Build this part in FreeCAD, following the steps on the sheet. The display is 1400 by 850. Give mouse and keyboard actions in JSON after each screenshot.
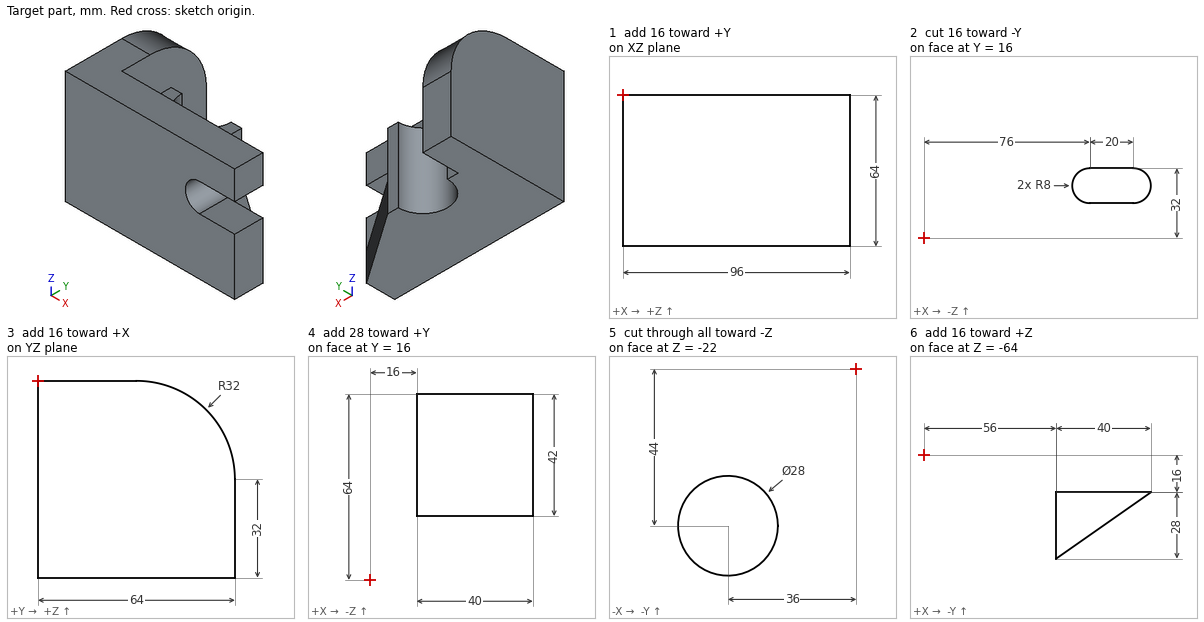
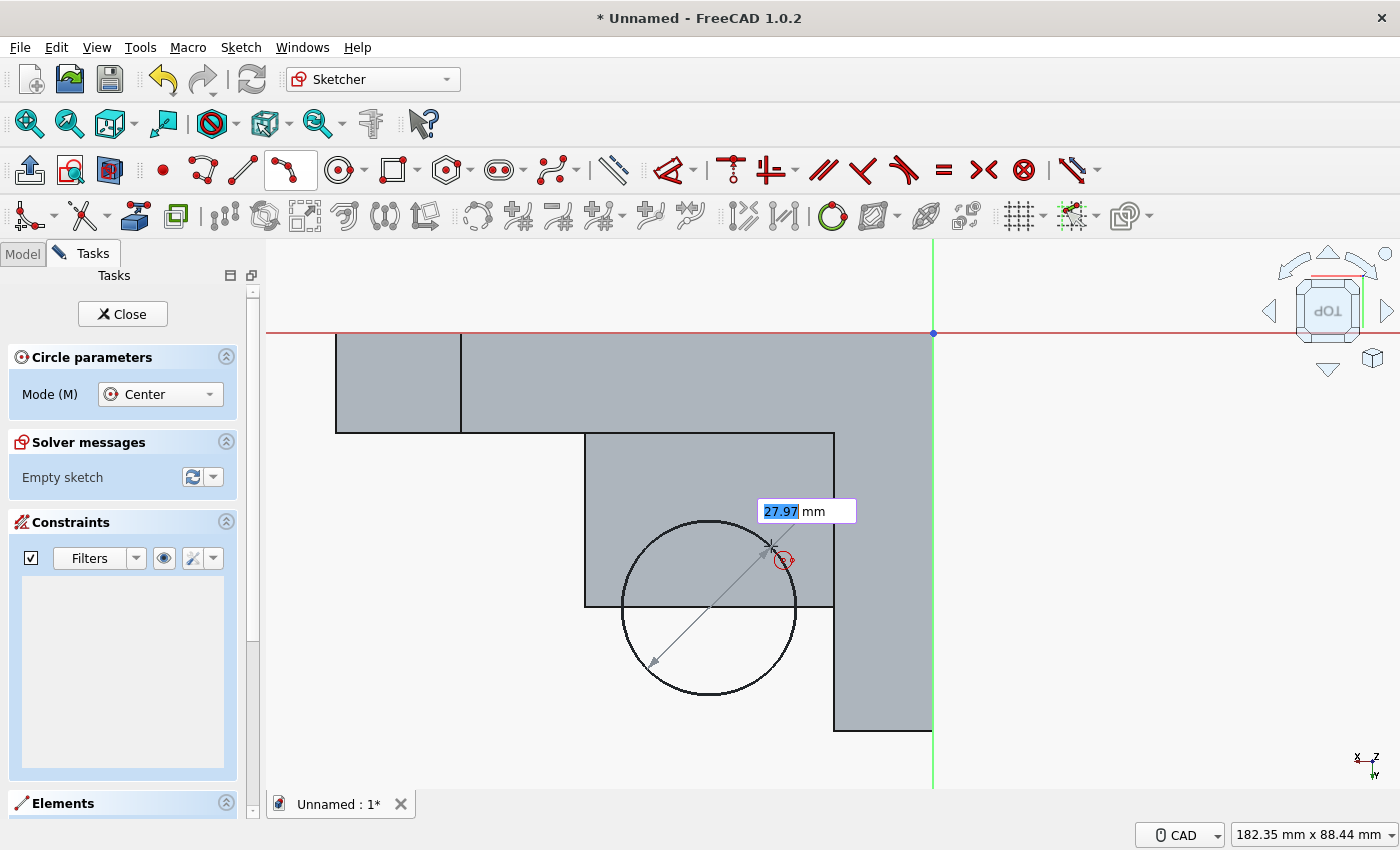
{"action": "type", "text": "28"}
{"action": "key", "text": "Return"}
{"action": "key", "text": "Escape"}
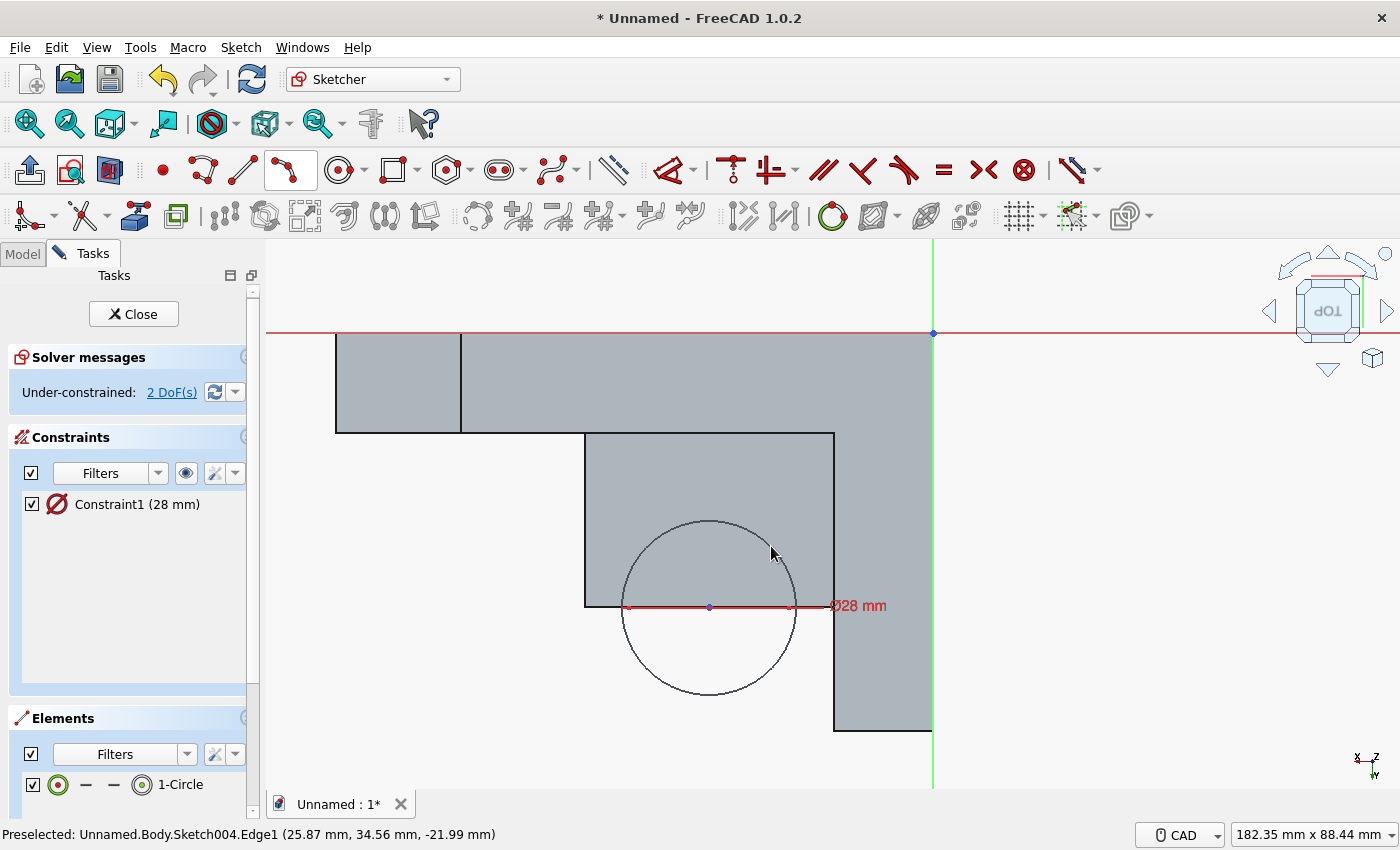
{"action": "key", "text": "d"}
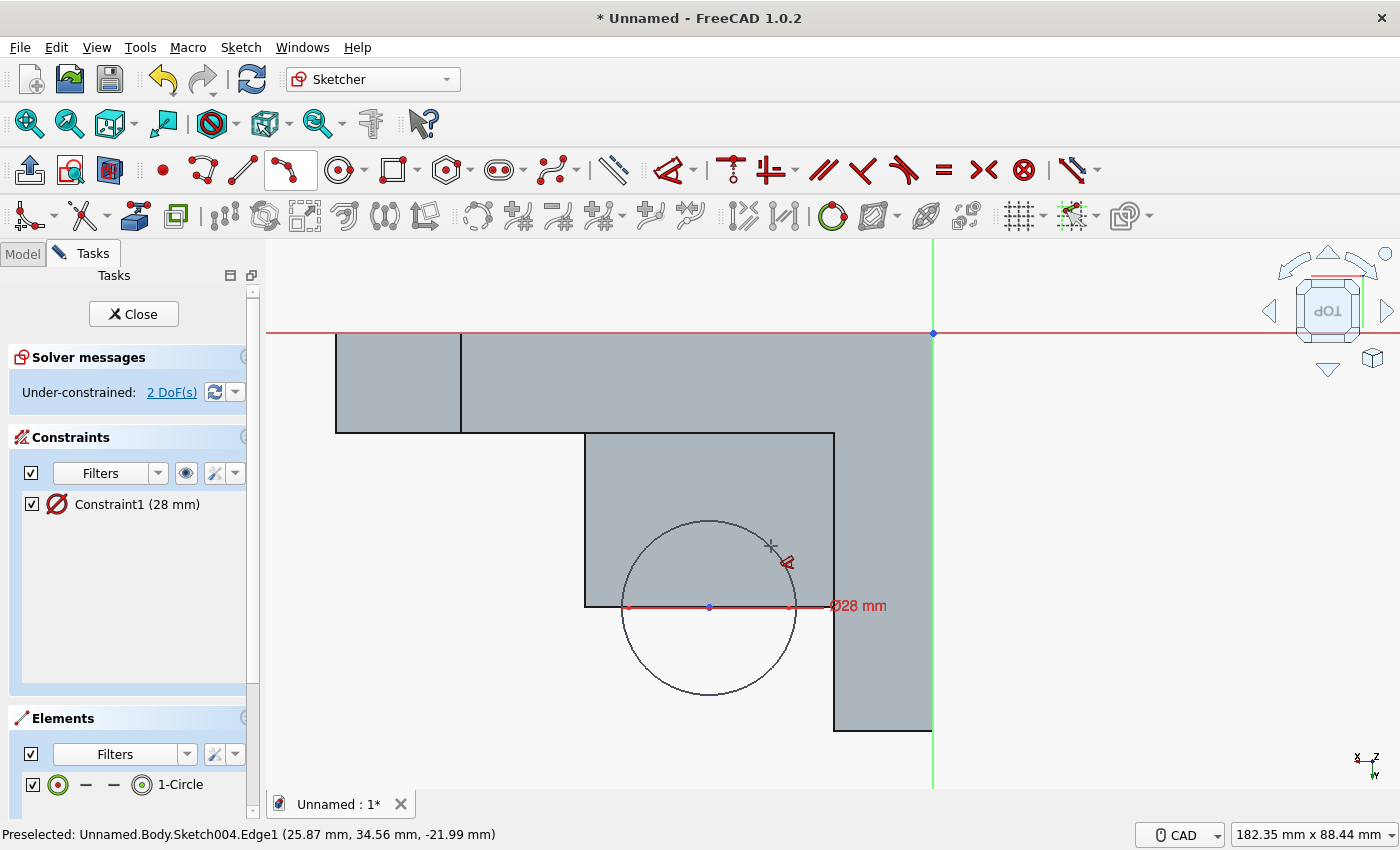
{"action": "left_click", "coordinate": [709, 608]}
{"action": "left_click", "coordinate": [821, 299]}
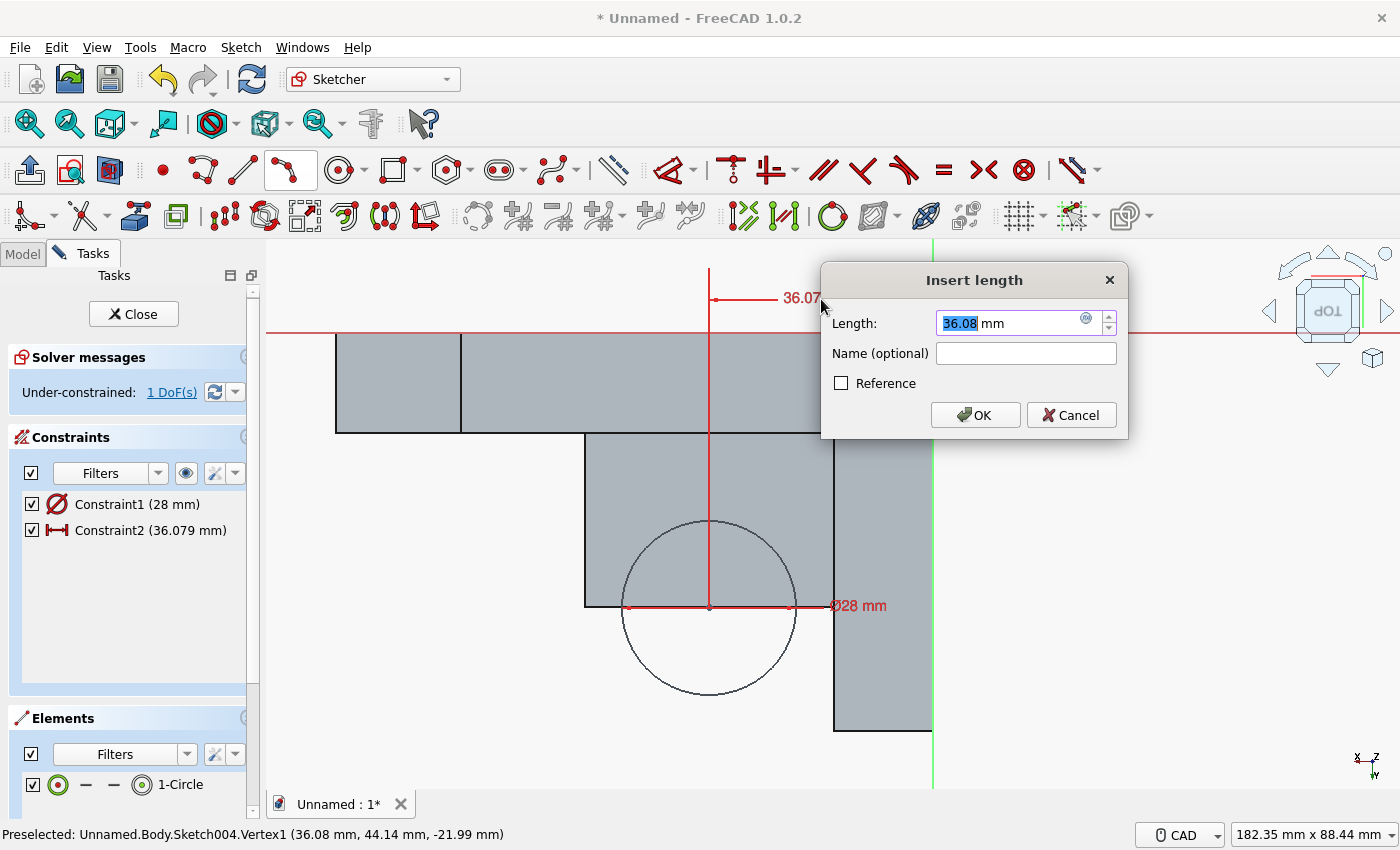
{"action": "type", "text": "36"}
{"action": "key", "text": "Return"}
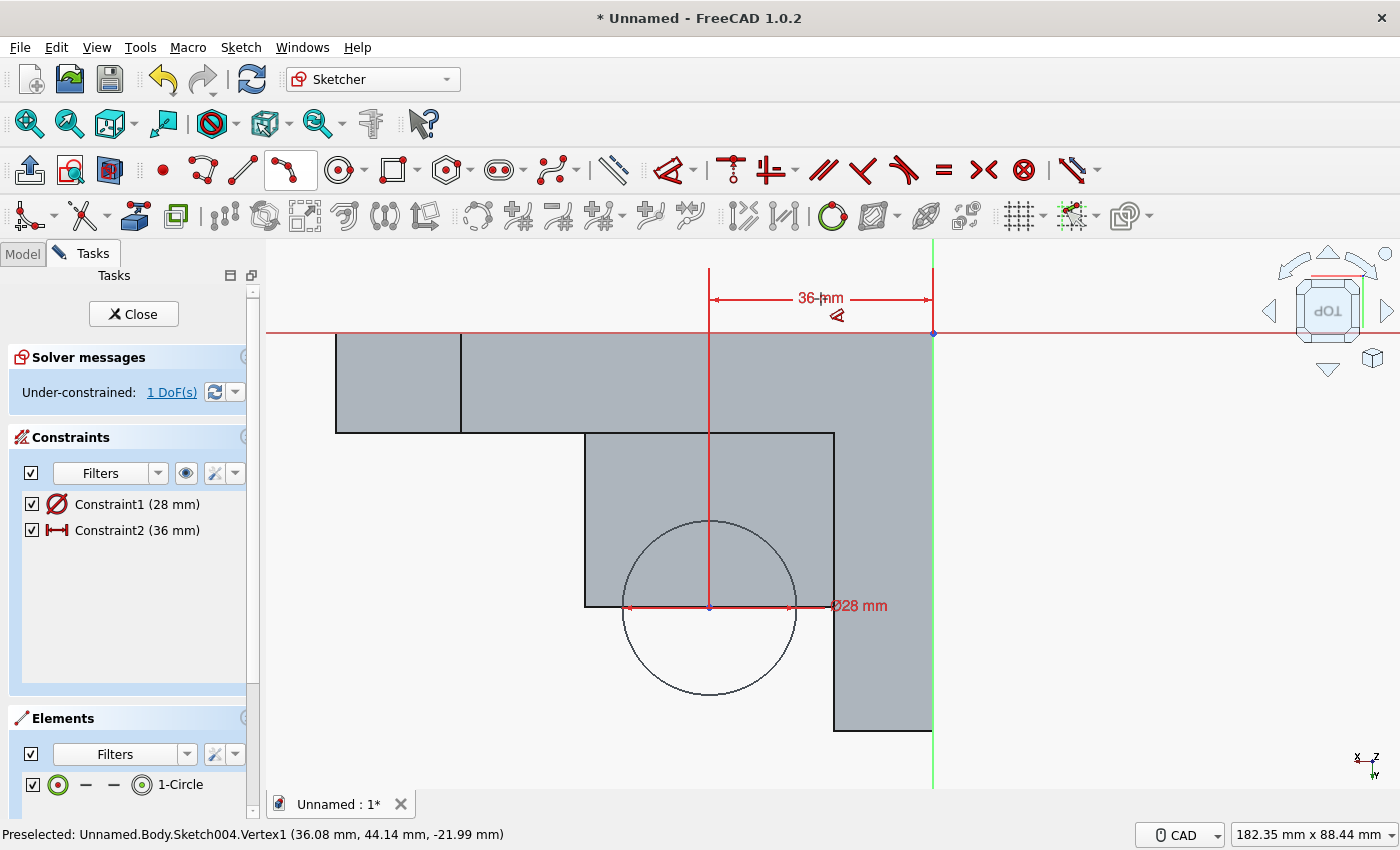
{"action": "left_click", "coordinate": [709, 608]}
{"action": "left_click", "coordinate": [967, 471]}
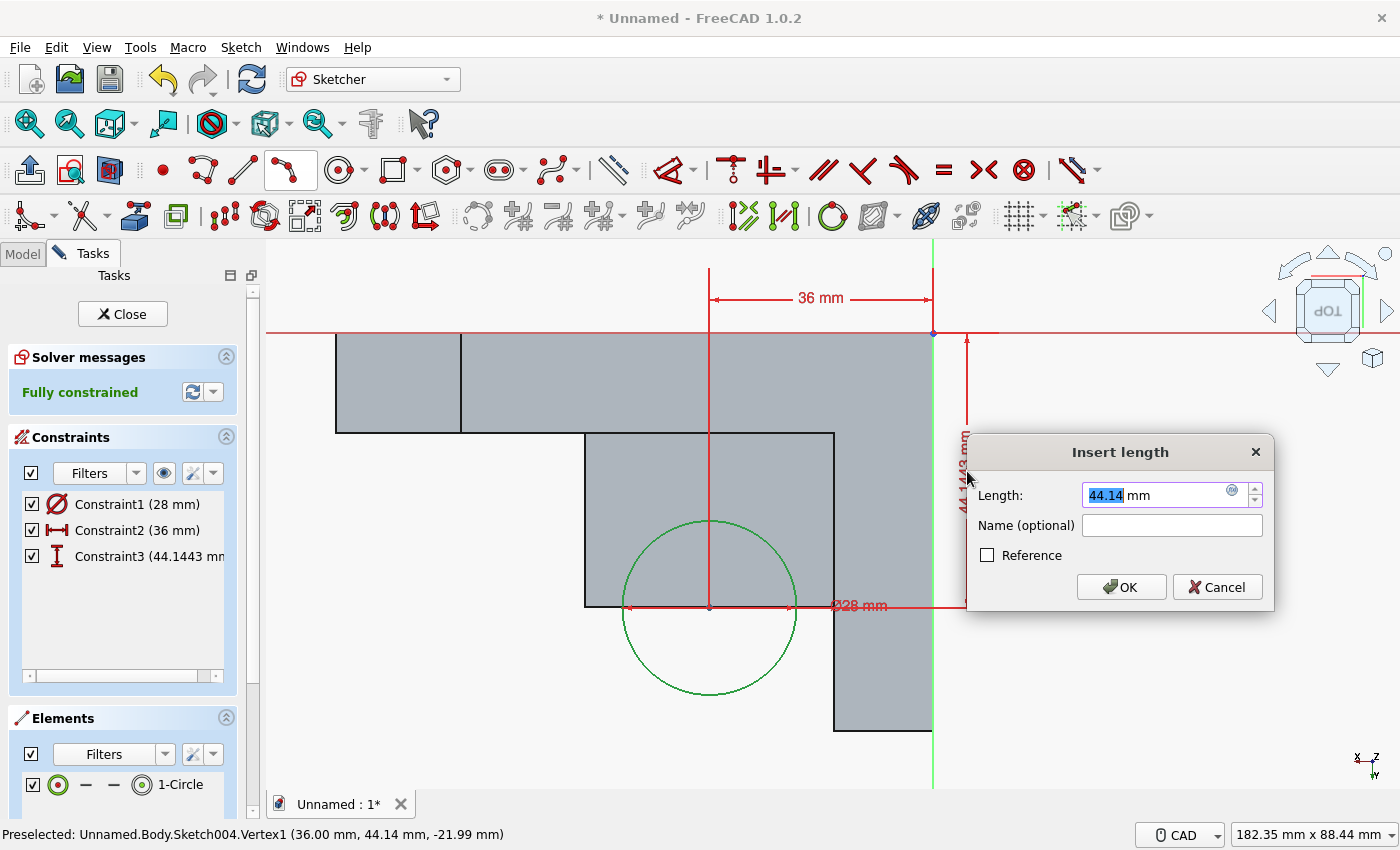
{"action": "type", "text": "44"}
{"action": "key", "text": "Return"}
{"action": "key", "text": "Escape"}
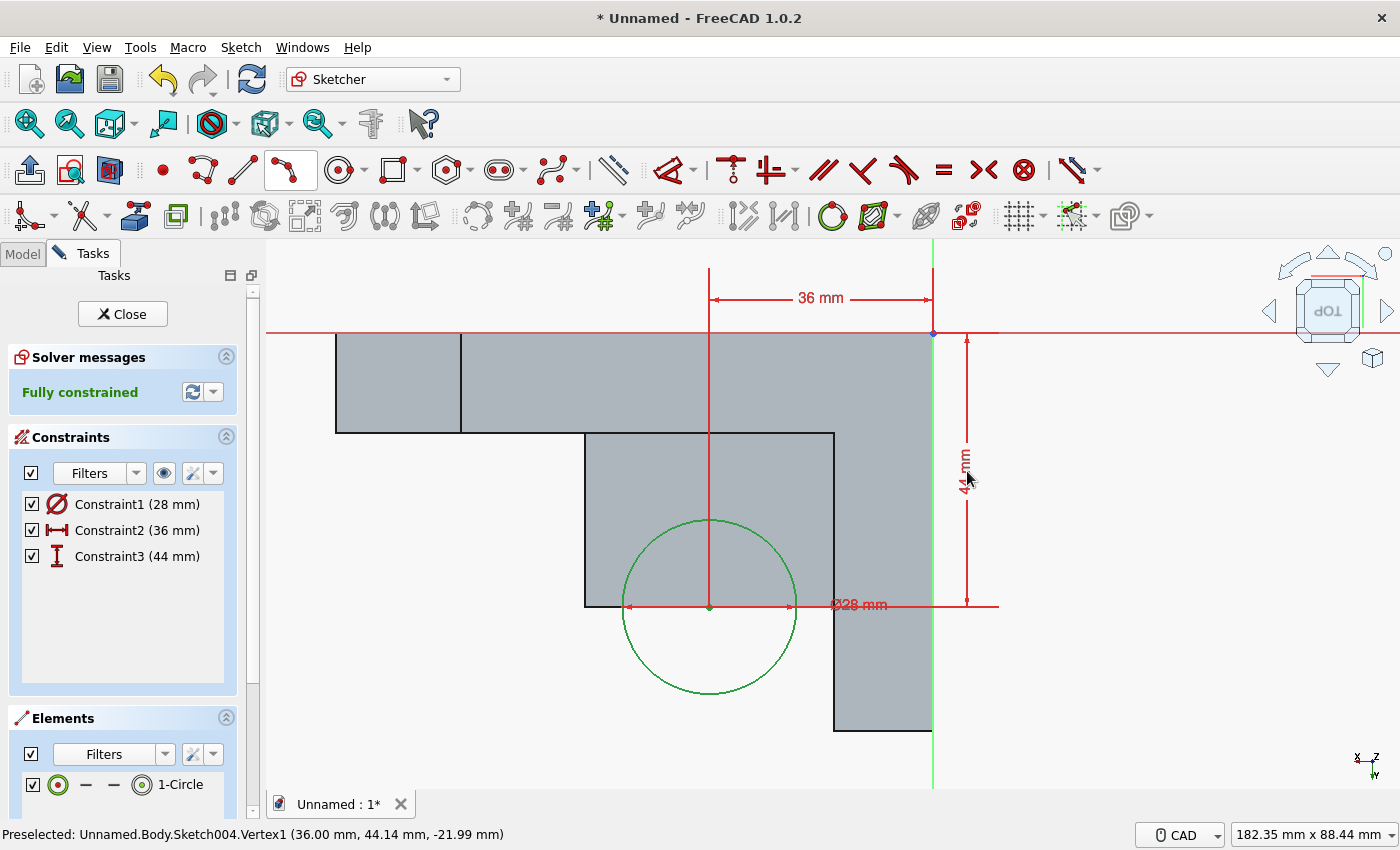
{"action": "left_click", "coordinate": [123, 314]}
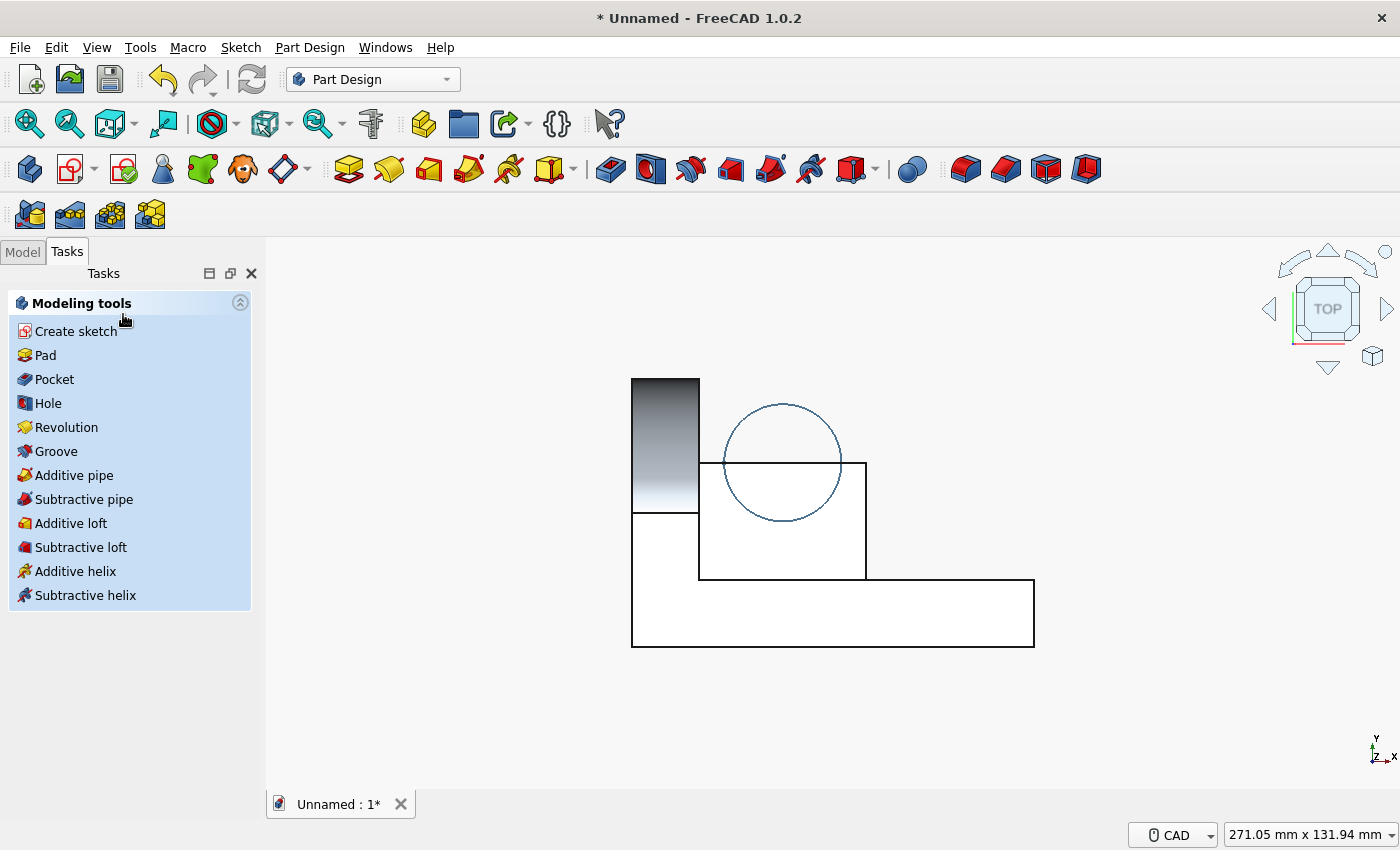
{"action": "left_click", "coordinate": [612, 170]}